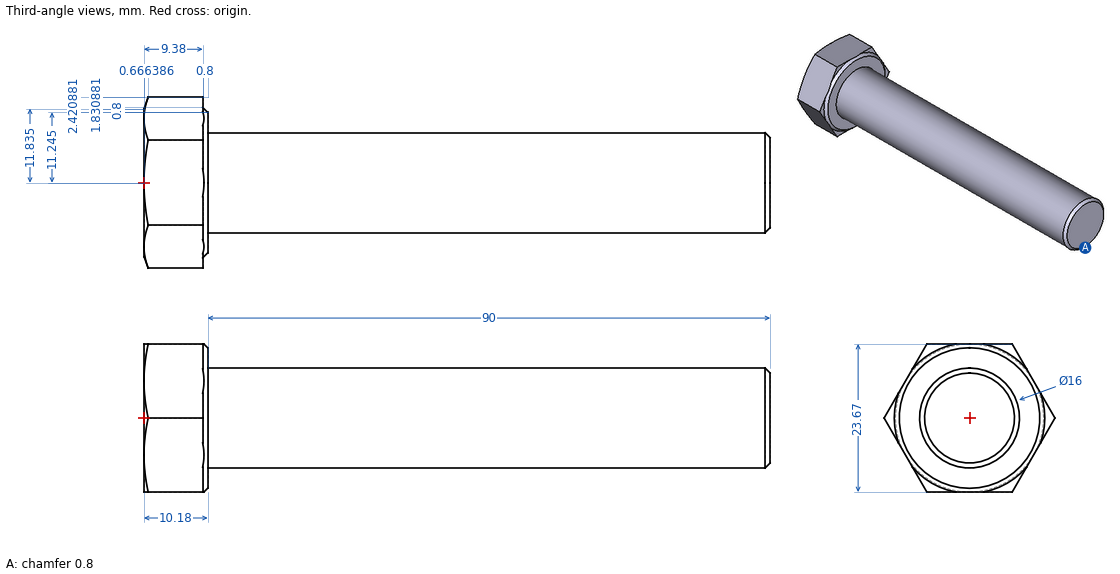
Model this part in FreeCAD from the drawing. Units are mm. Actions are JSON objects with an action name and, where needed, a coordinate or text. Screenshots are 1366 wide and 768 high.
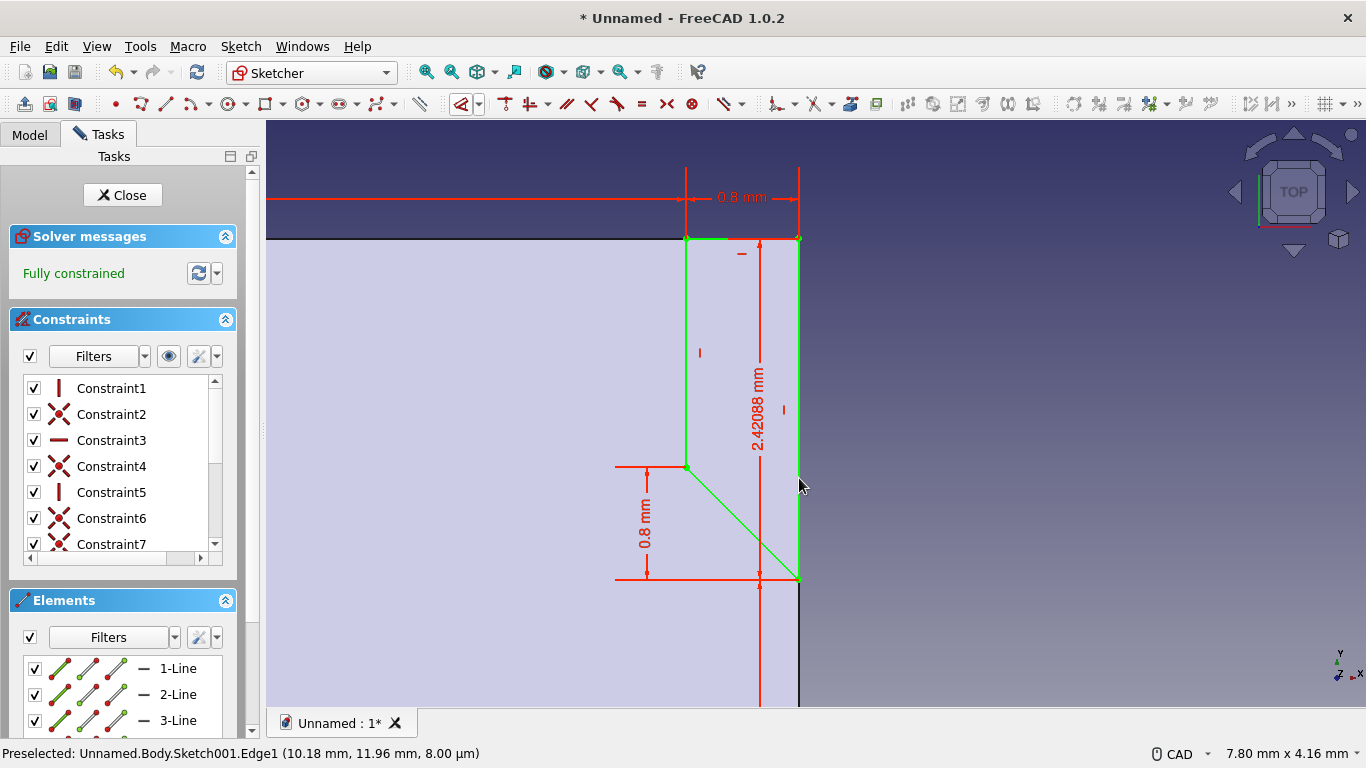
{"action": "left_click", "coordinate": [123, 195]}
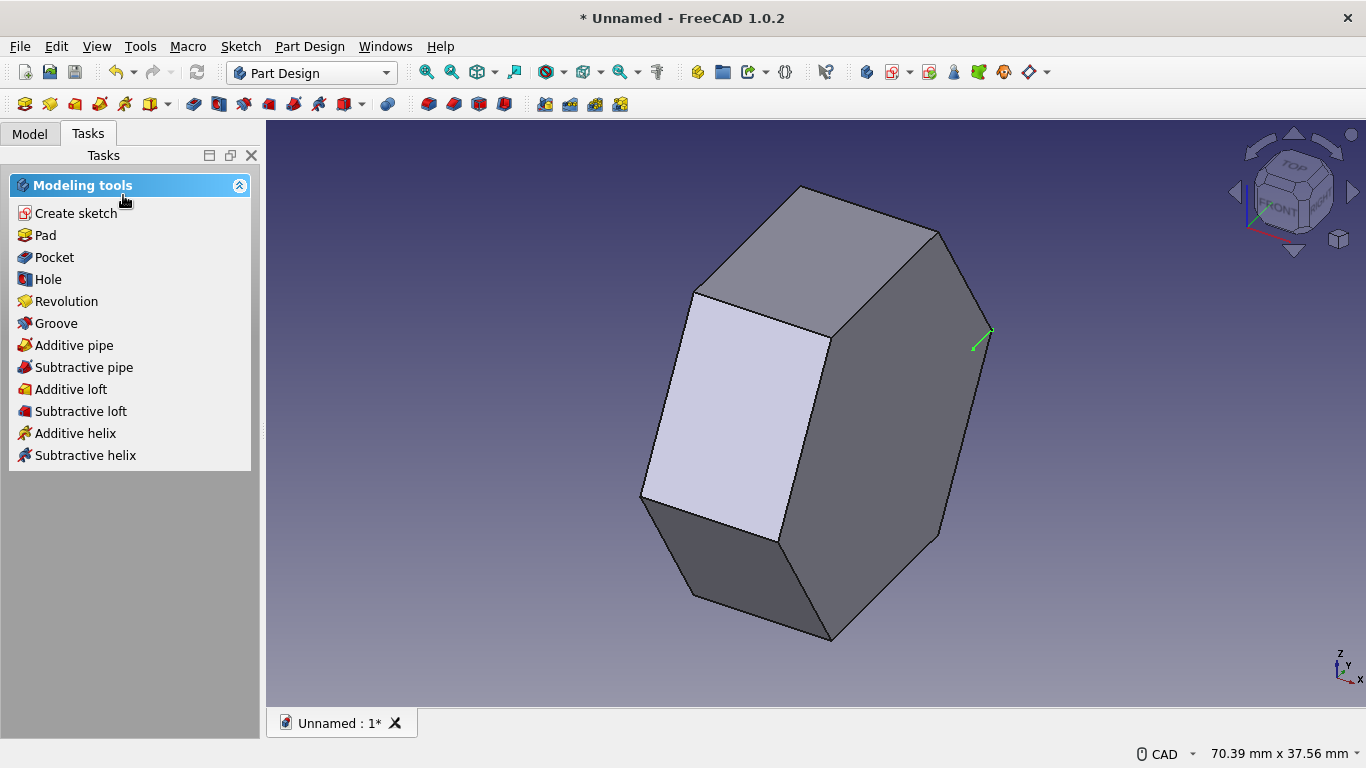
{"action": "left_click", "coordinate": [244, 104]}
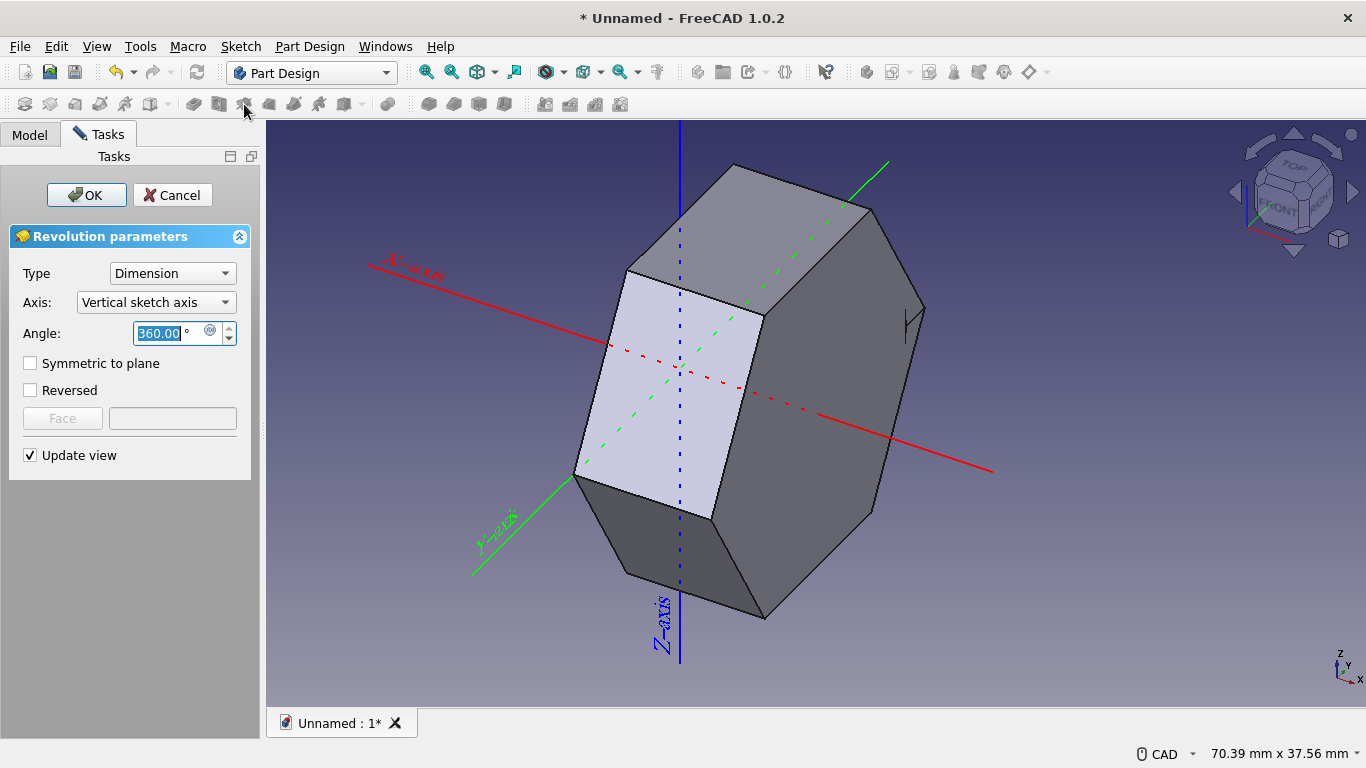
{"action": "left_click", "coordinate": [157, 302]}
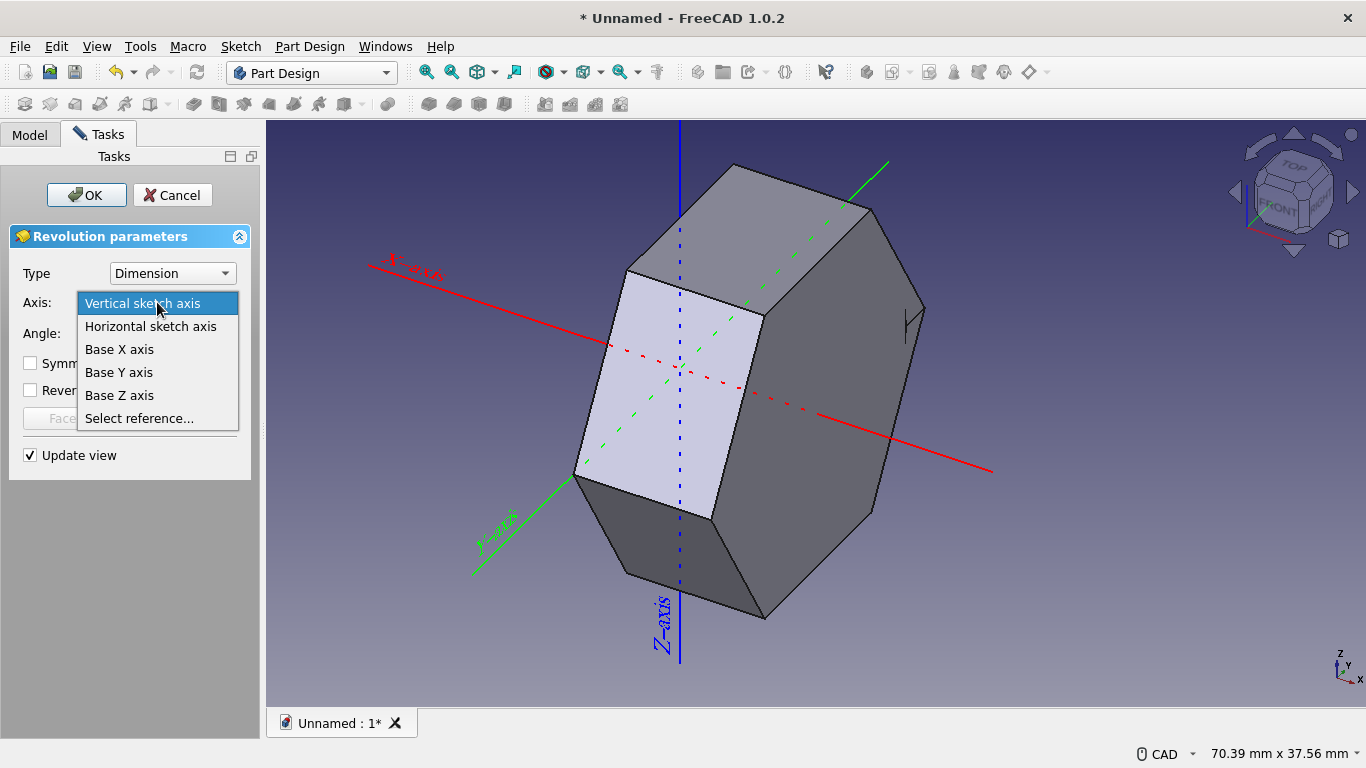
{"action": "left_click", "coordinate": [156, 326]}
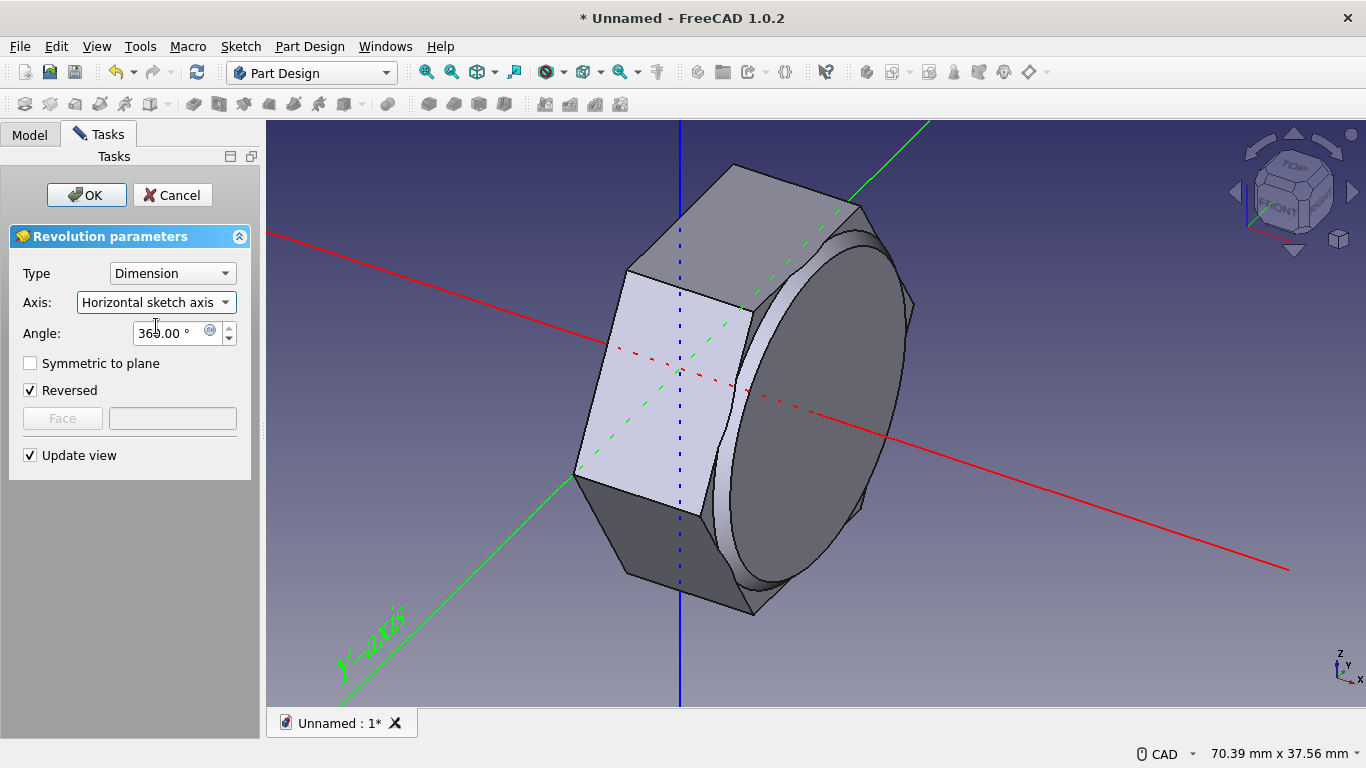
{"action": "left_click", "coordinate": [87, 195]}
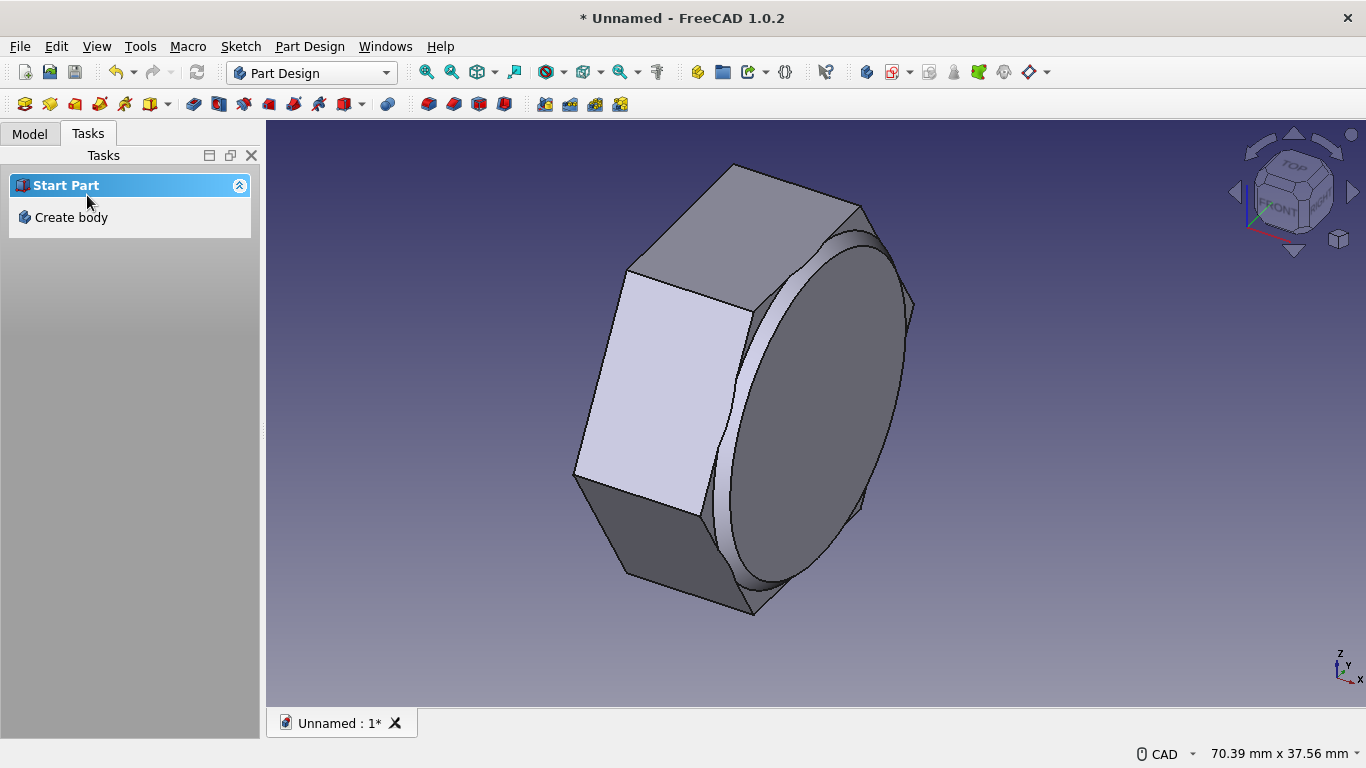
{"action": "key", "text": "v f"}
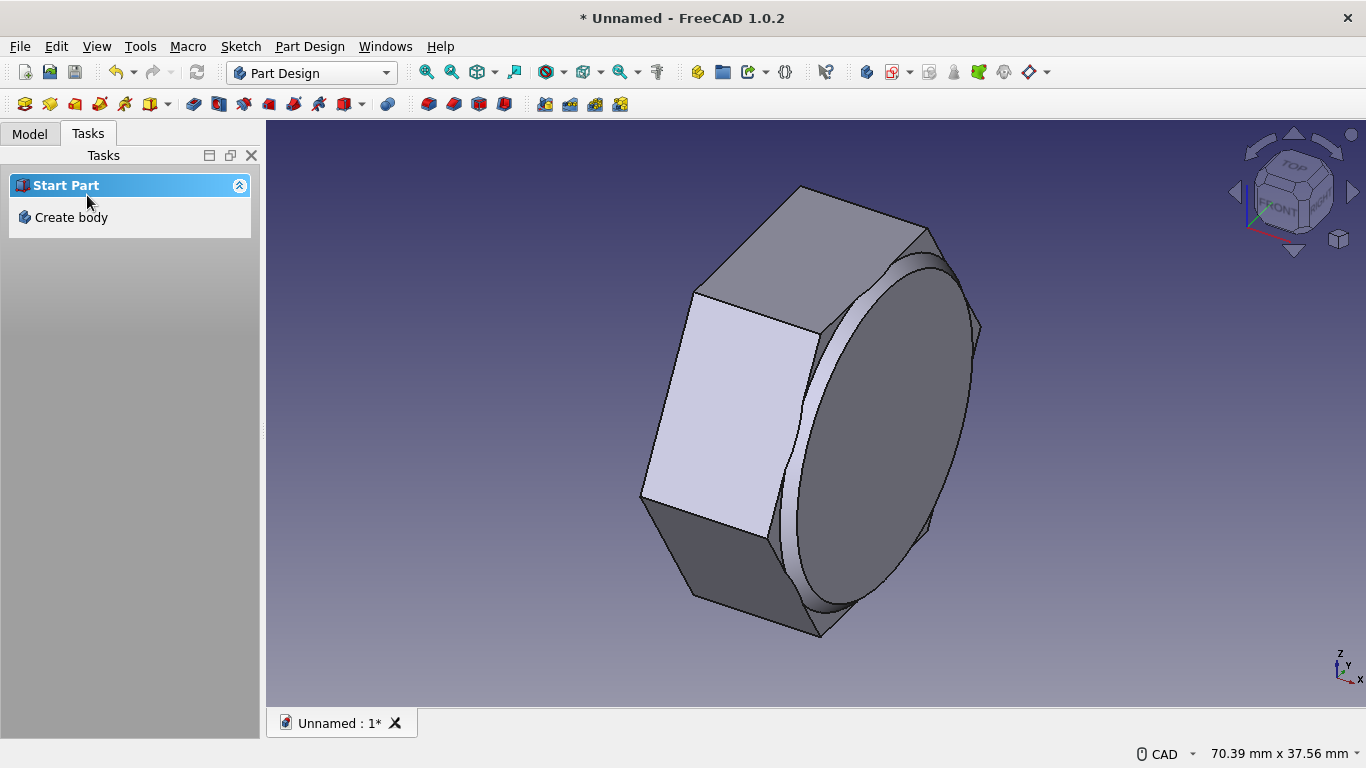
{"action": "left_click", "coordinate": [892, 72]}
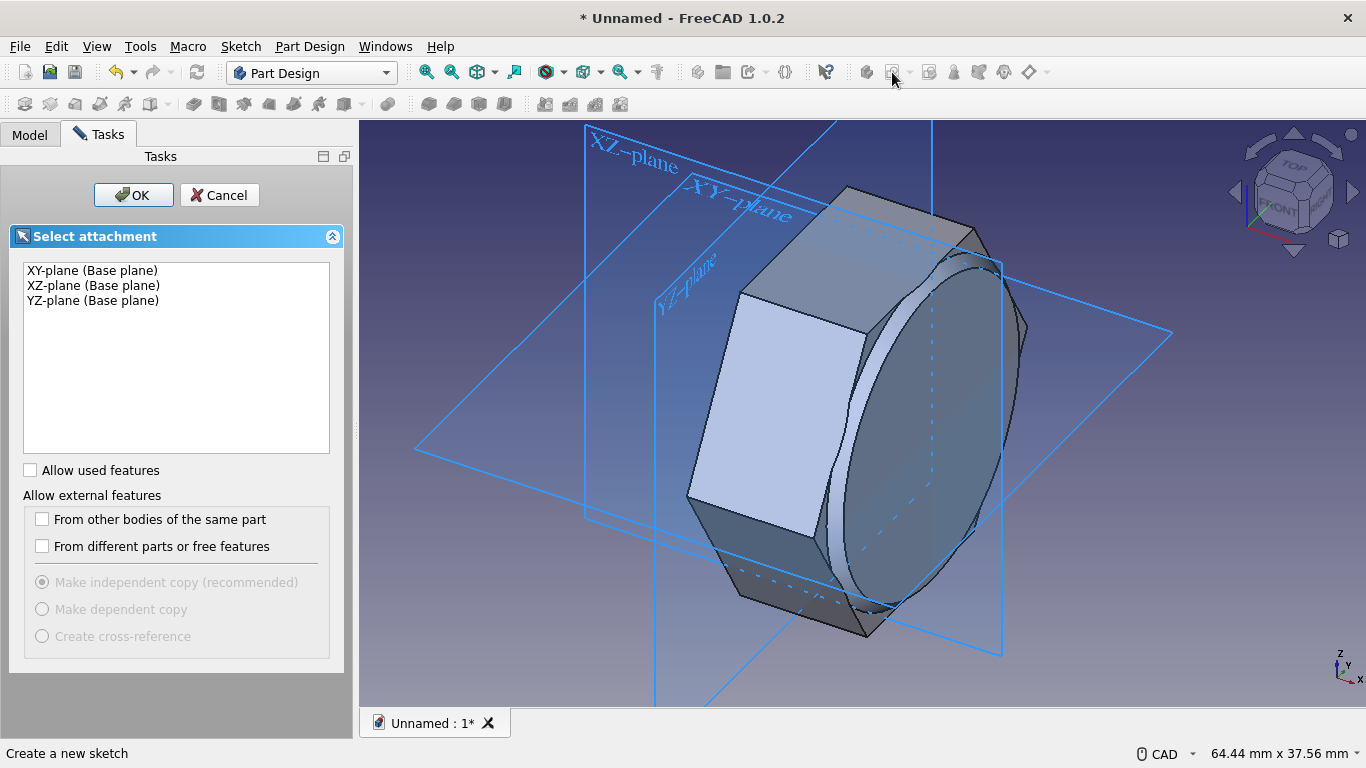
{"action": "left_click", "coordinate": [84, 270]}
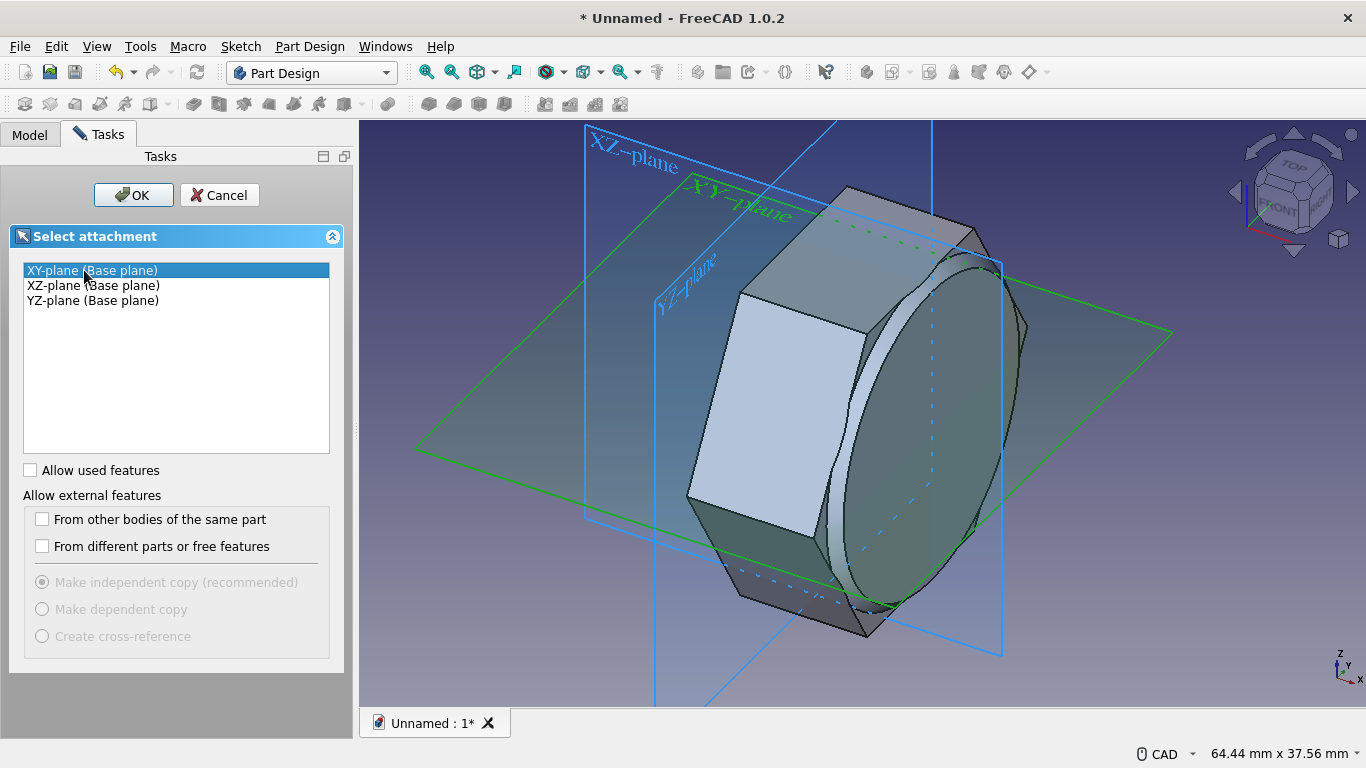
{"action": "left_click", "coordinate": [134, 195]}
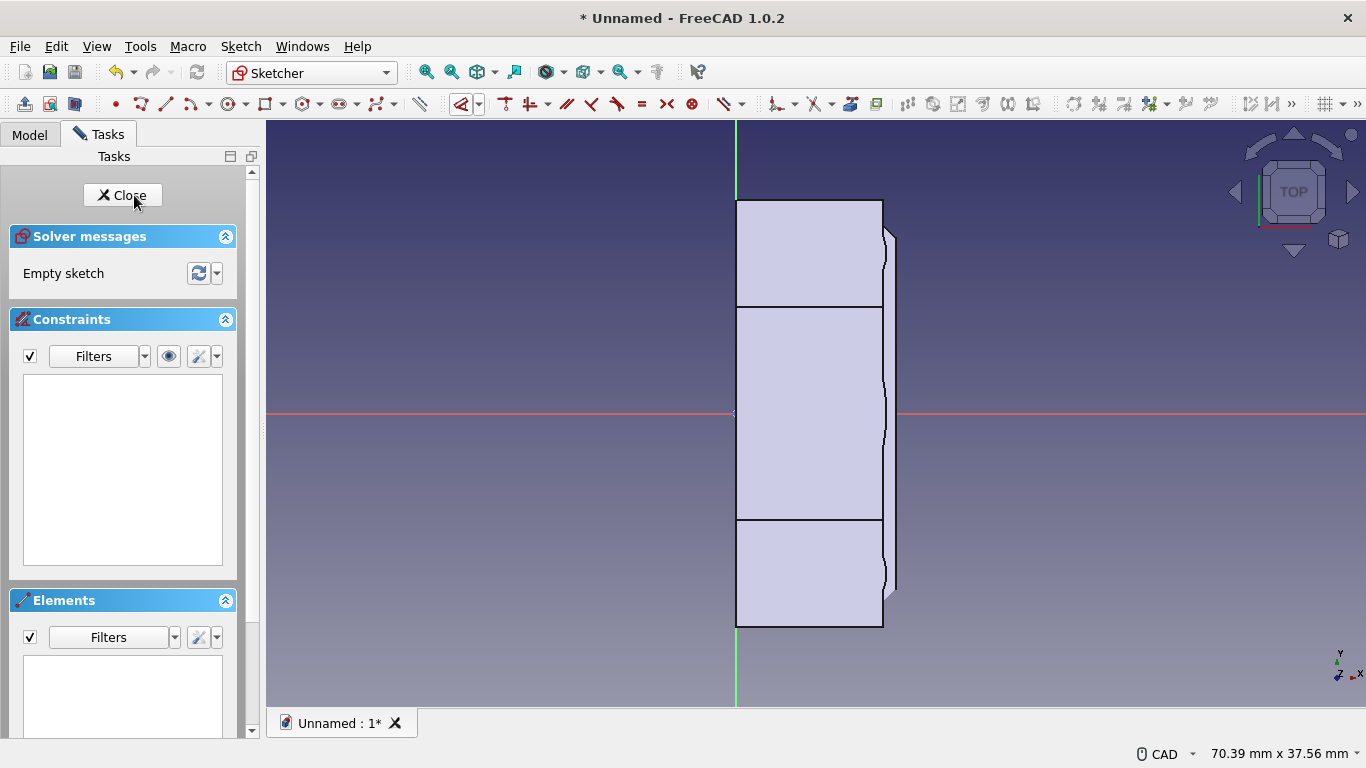
{"action": "key", "text": "q s"}